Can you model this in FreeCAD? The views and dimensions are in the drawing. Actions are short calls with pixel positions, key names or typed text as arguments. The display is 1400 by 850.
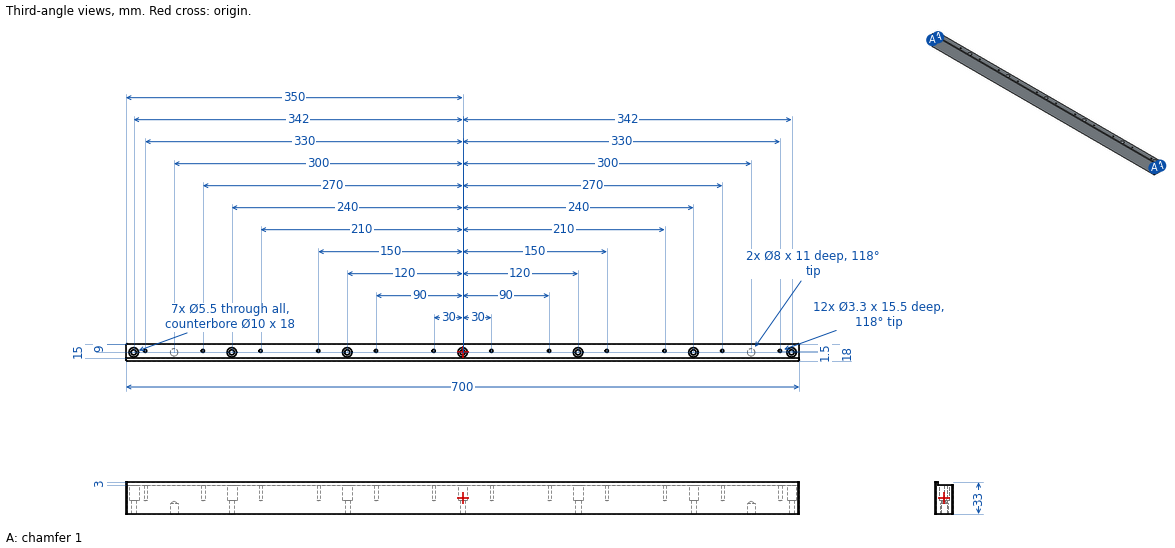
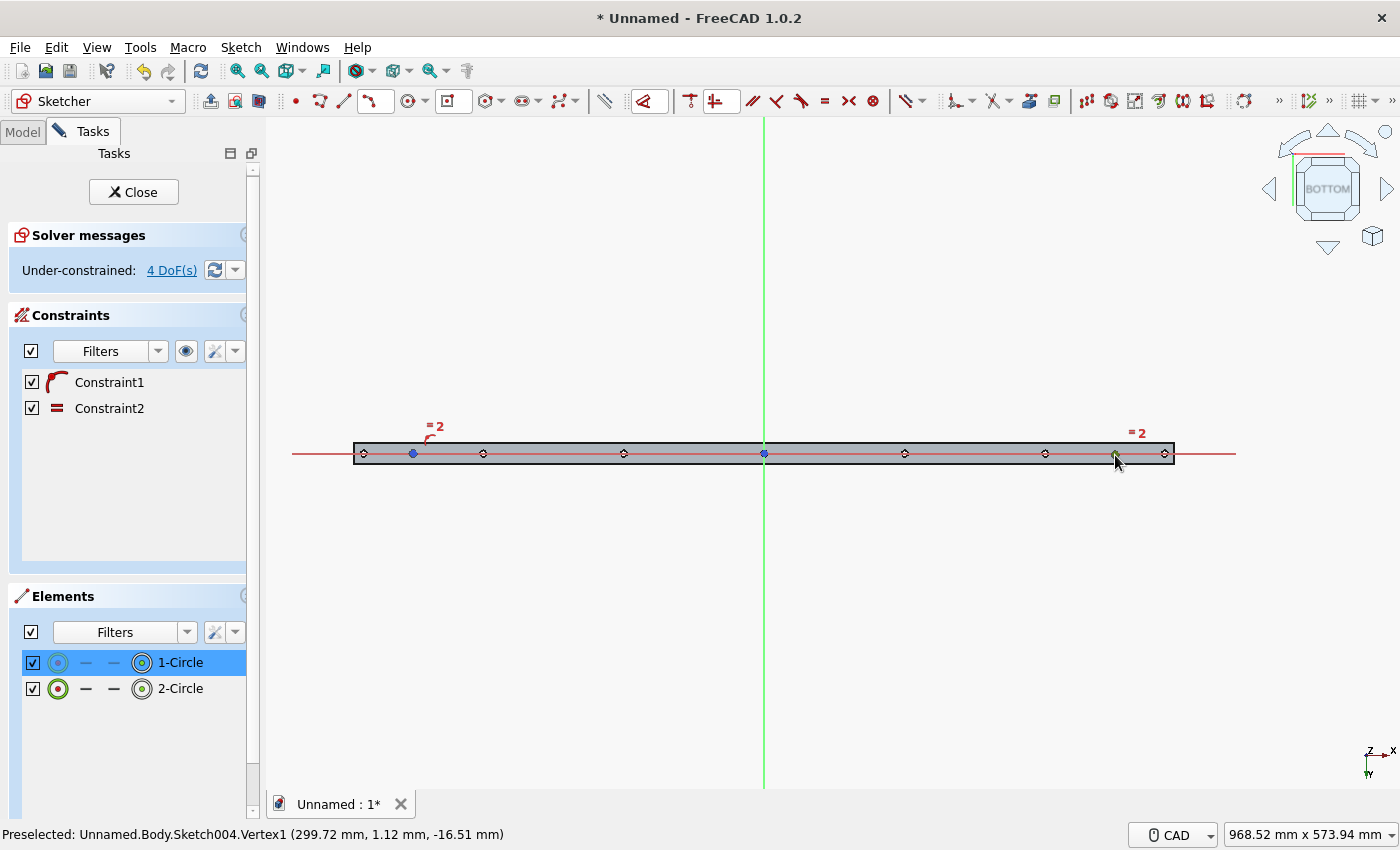
click(361, 454)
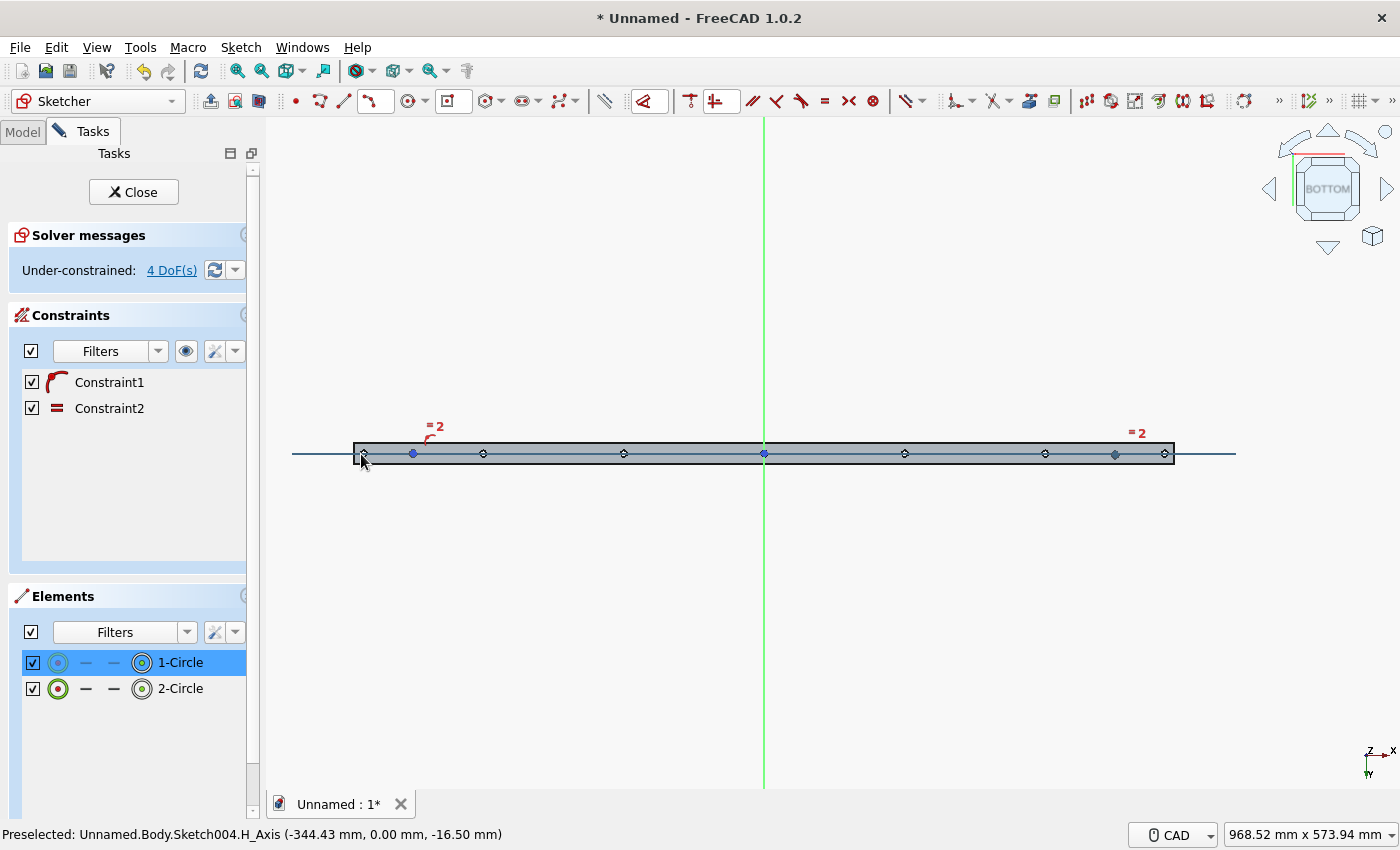
key(c)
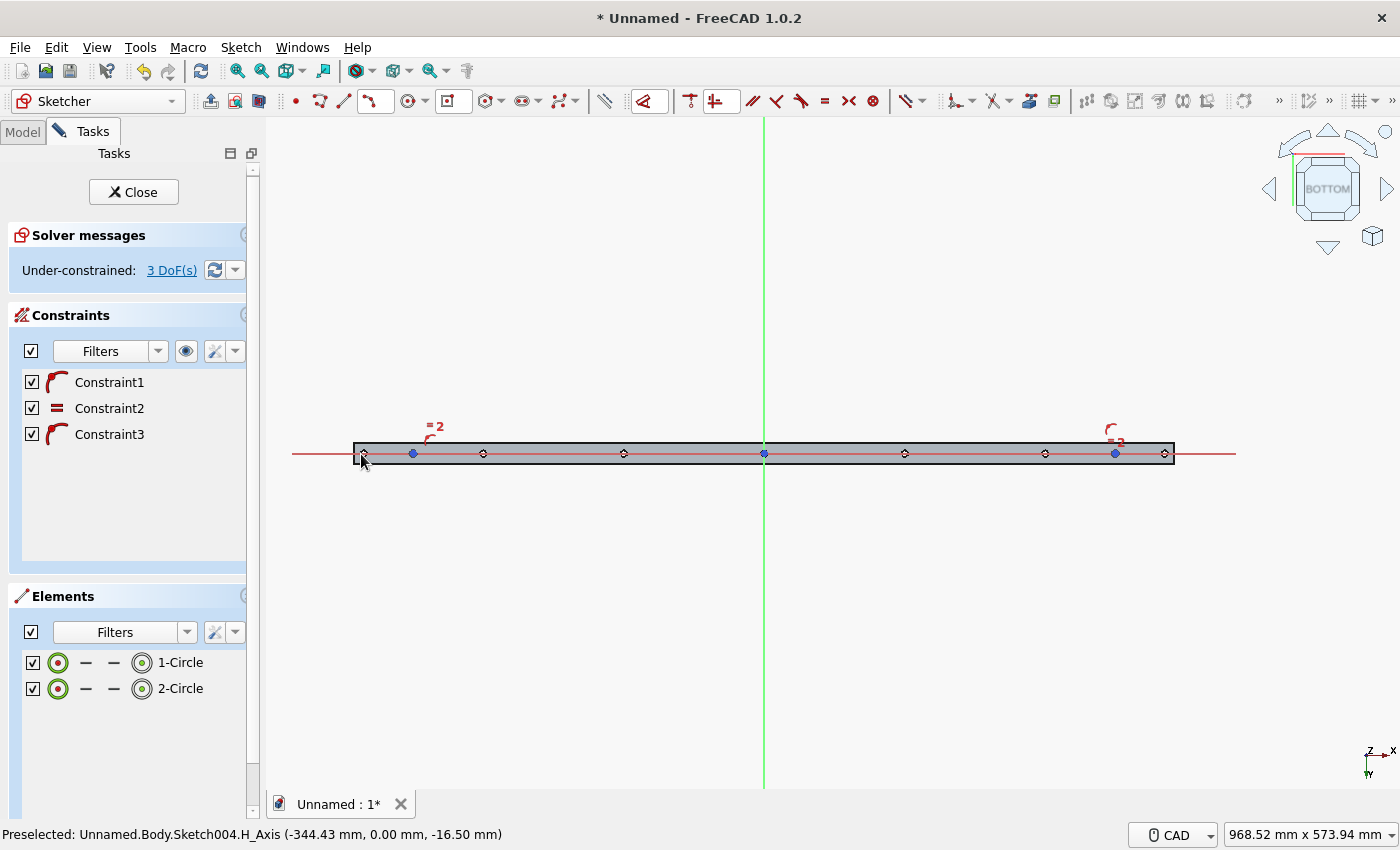
scroll(1112, 454, up, 8)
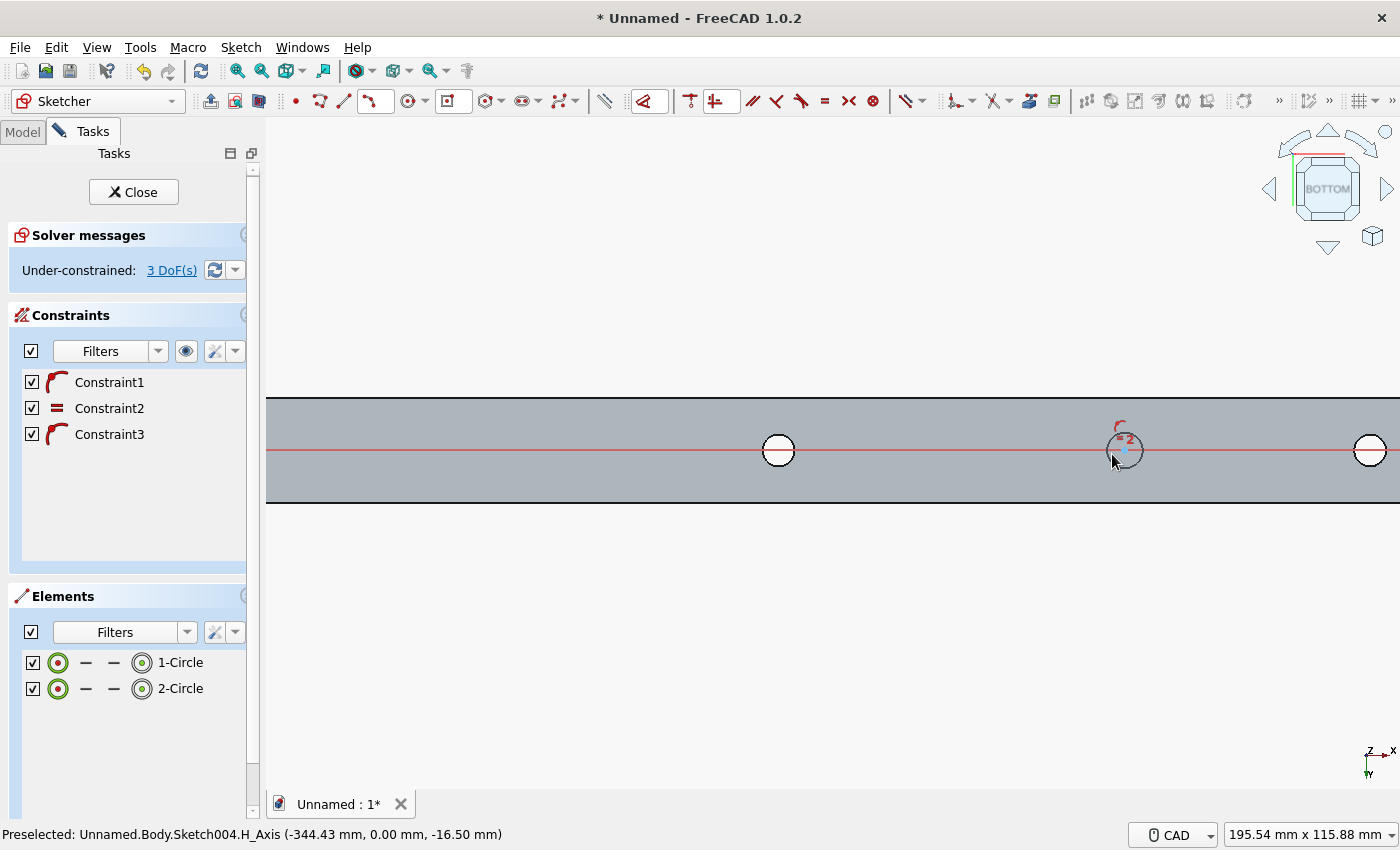
click(1107, 450)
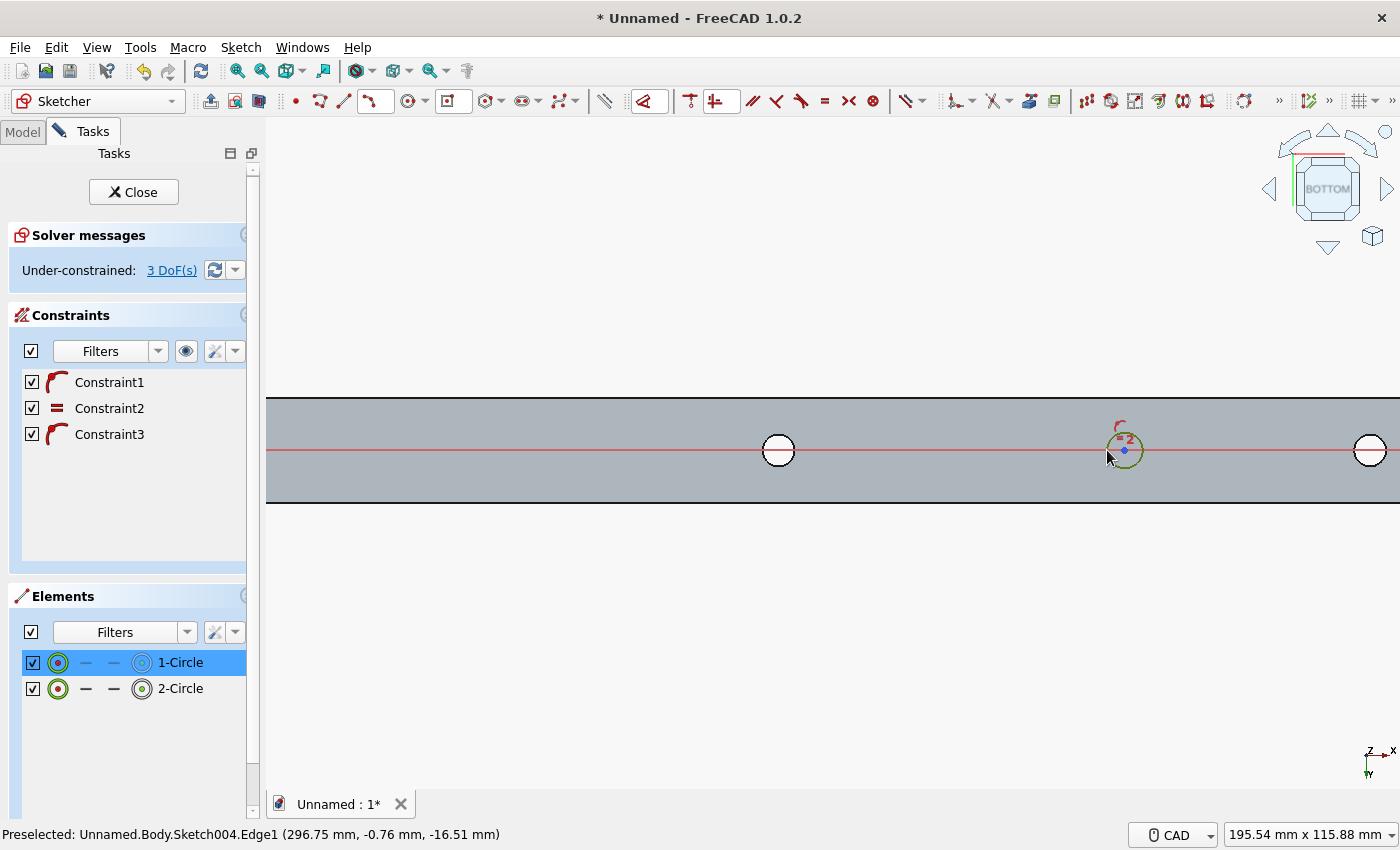
key(k)
key(o)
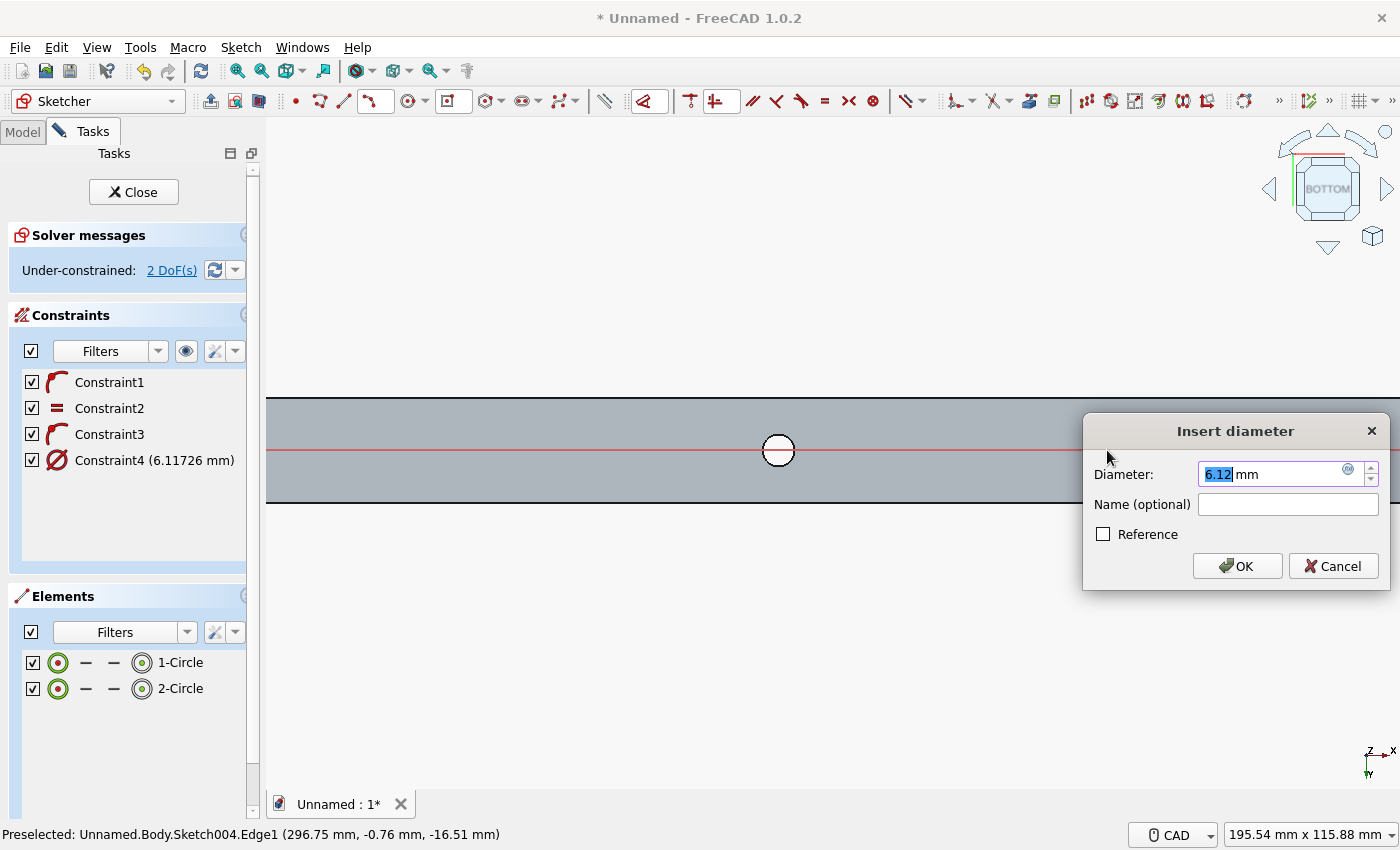
text(8)
key(Return)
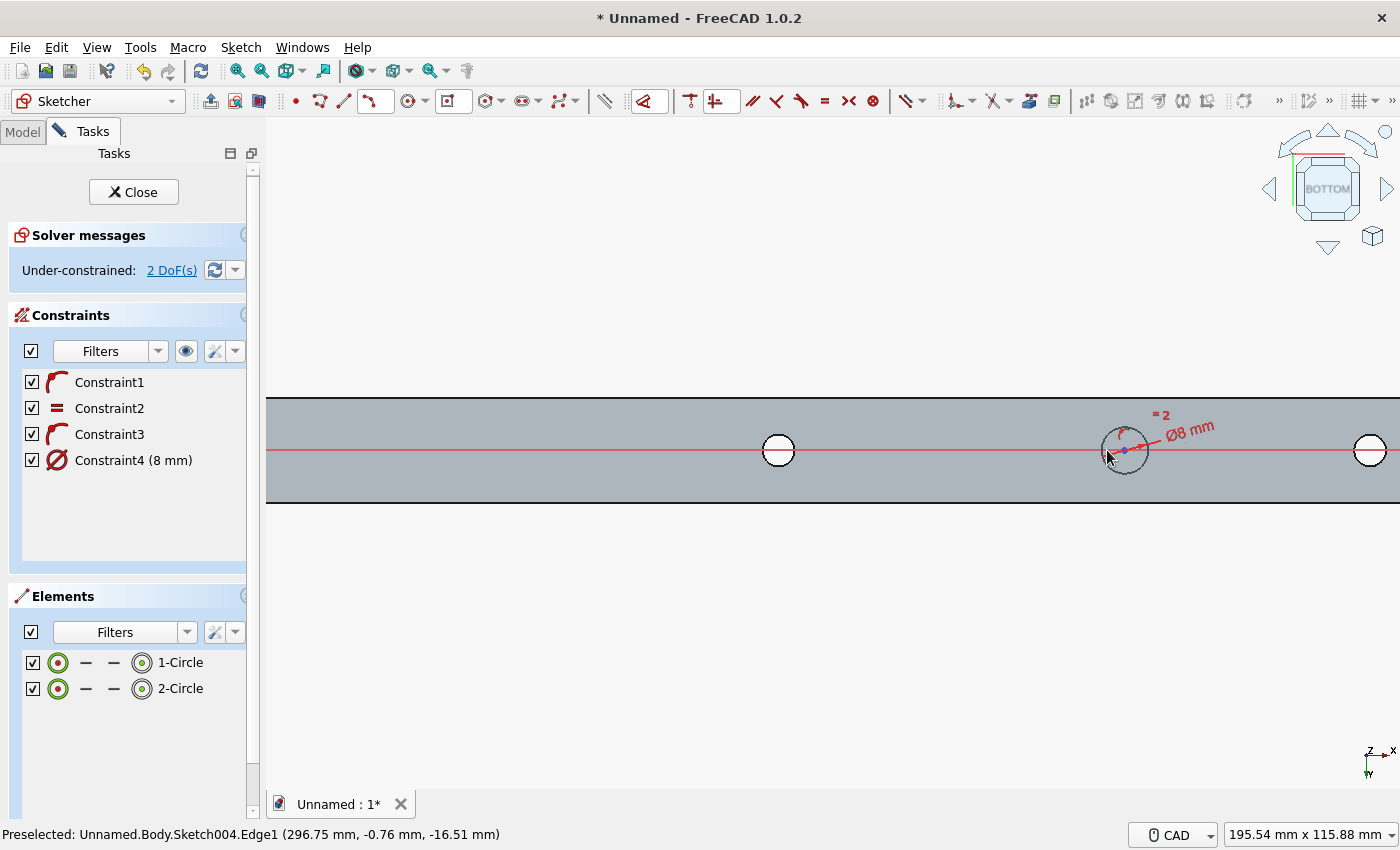
scroll(1113, 454, down, 8)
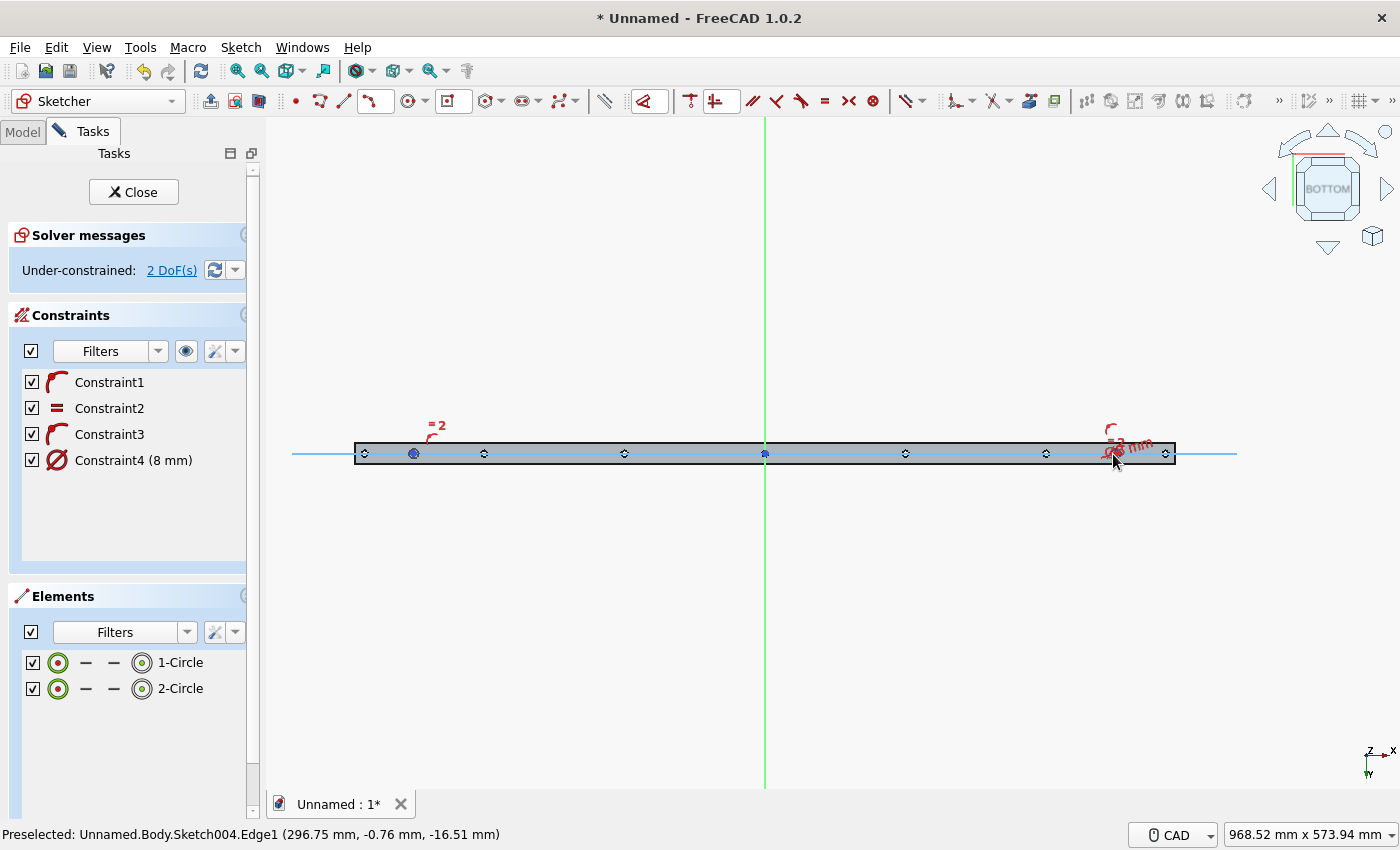
click(1116, 454)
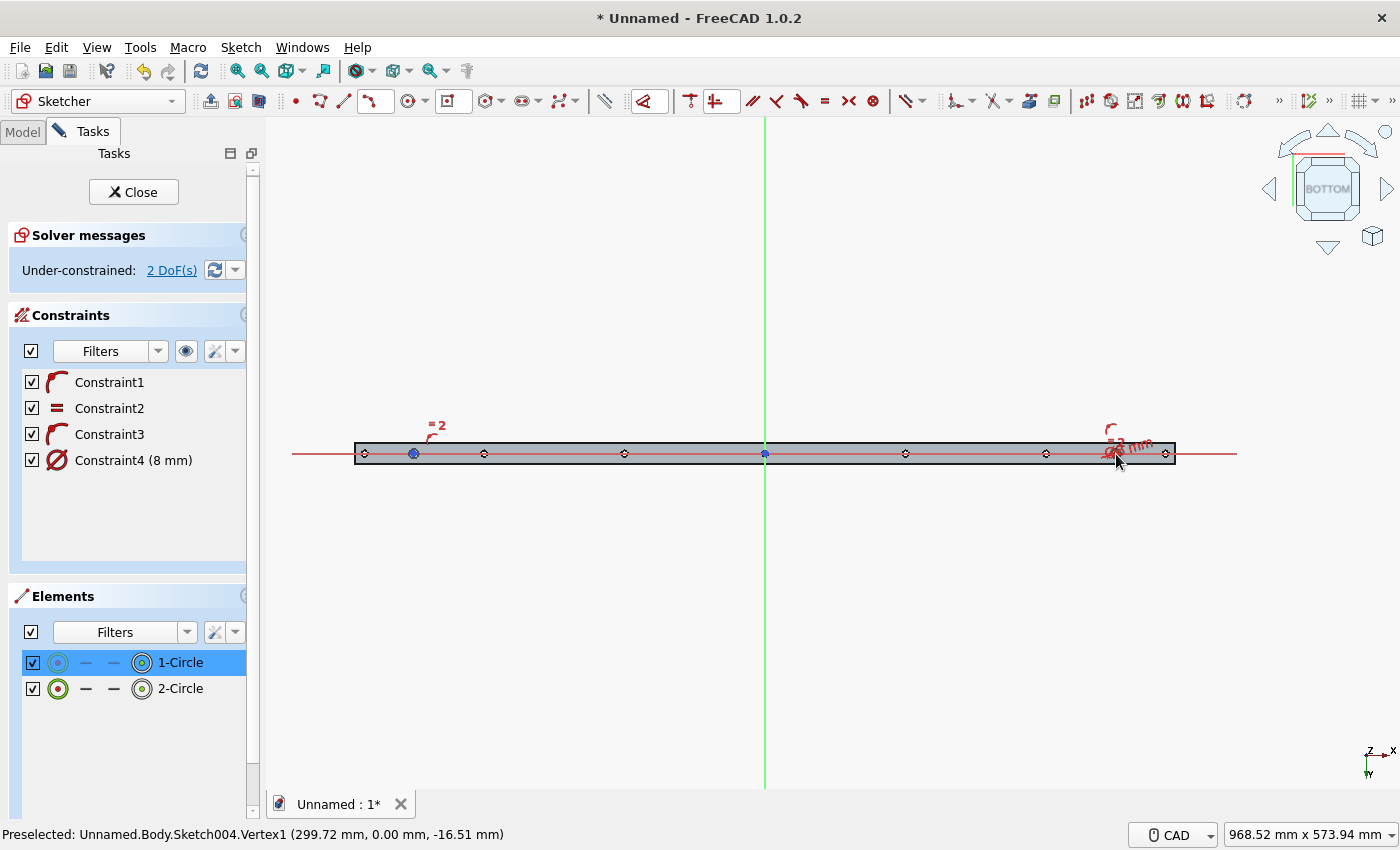
click(662, 102)